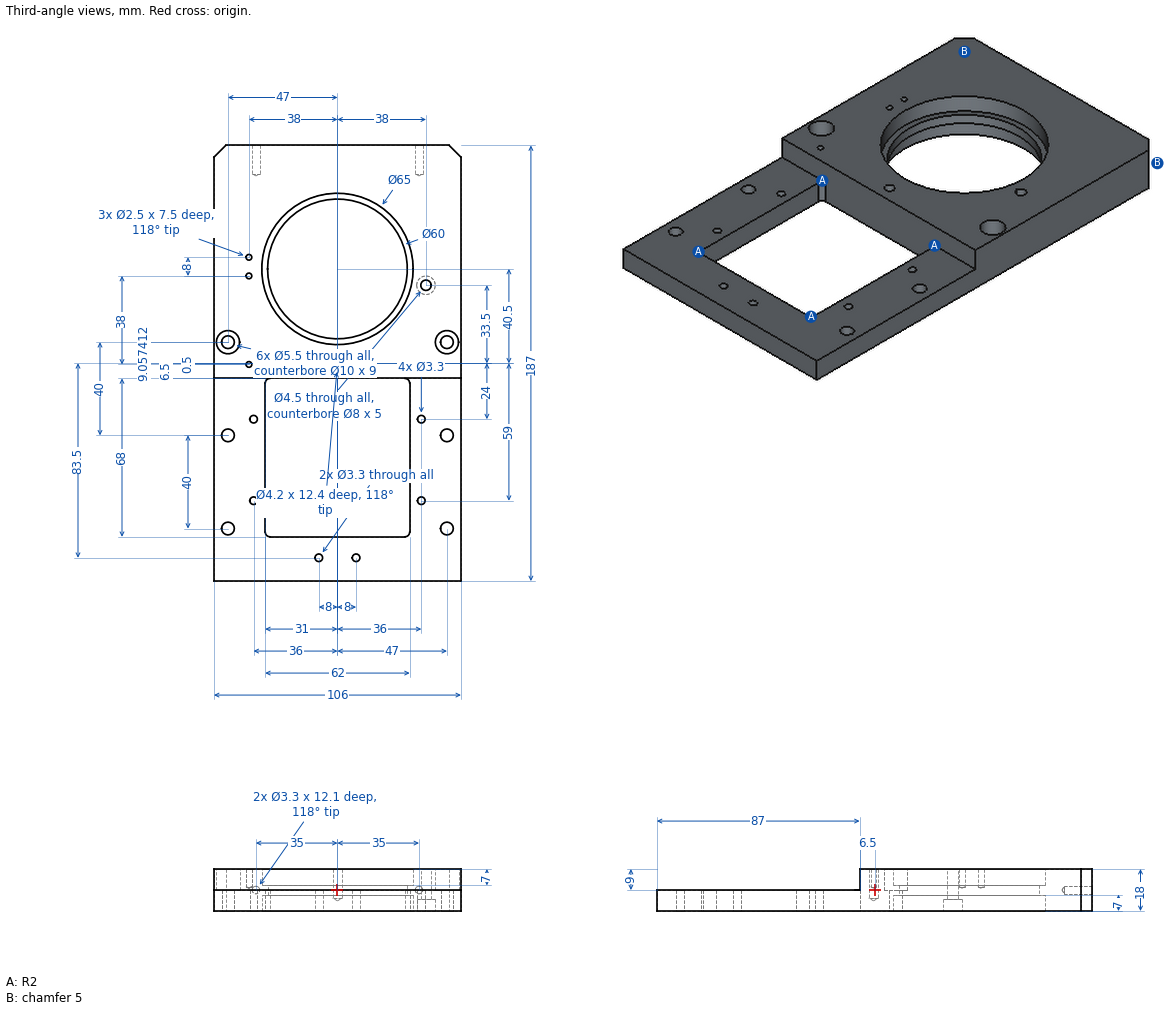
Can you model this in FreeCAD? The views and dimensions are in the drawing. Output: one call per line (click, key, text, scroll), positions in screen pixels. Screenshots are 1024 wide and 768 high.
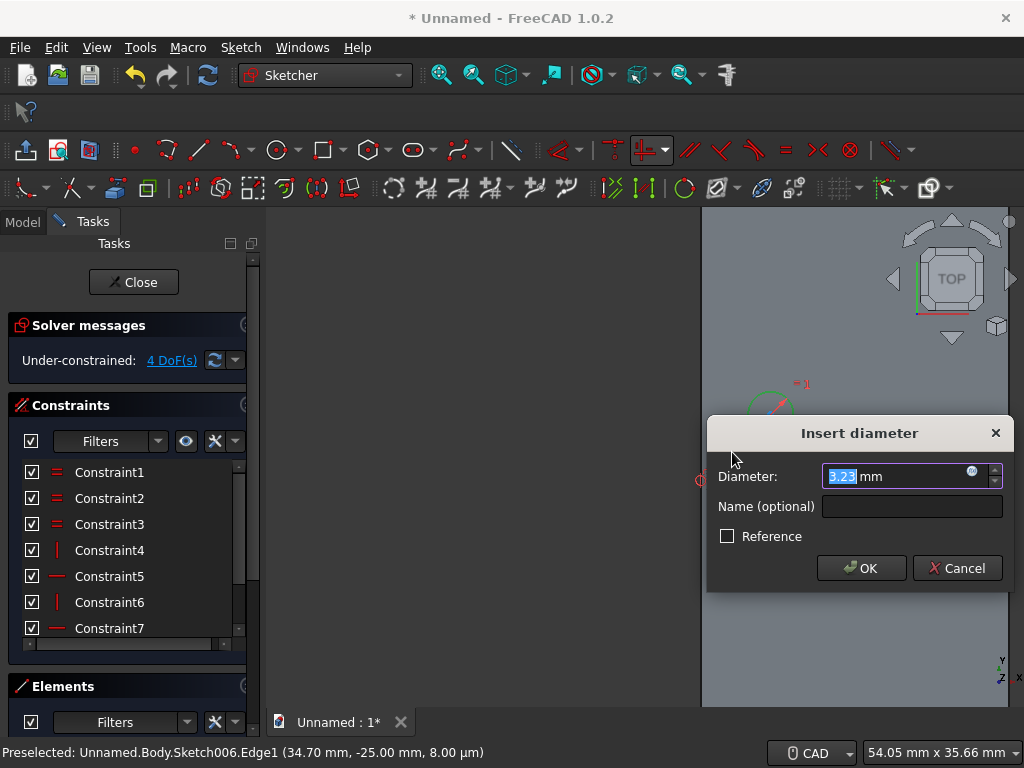
text(3.3)
key(Return)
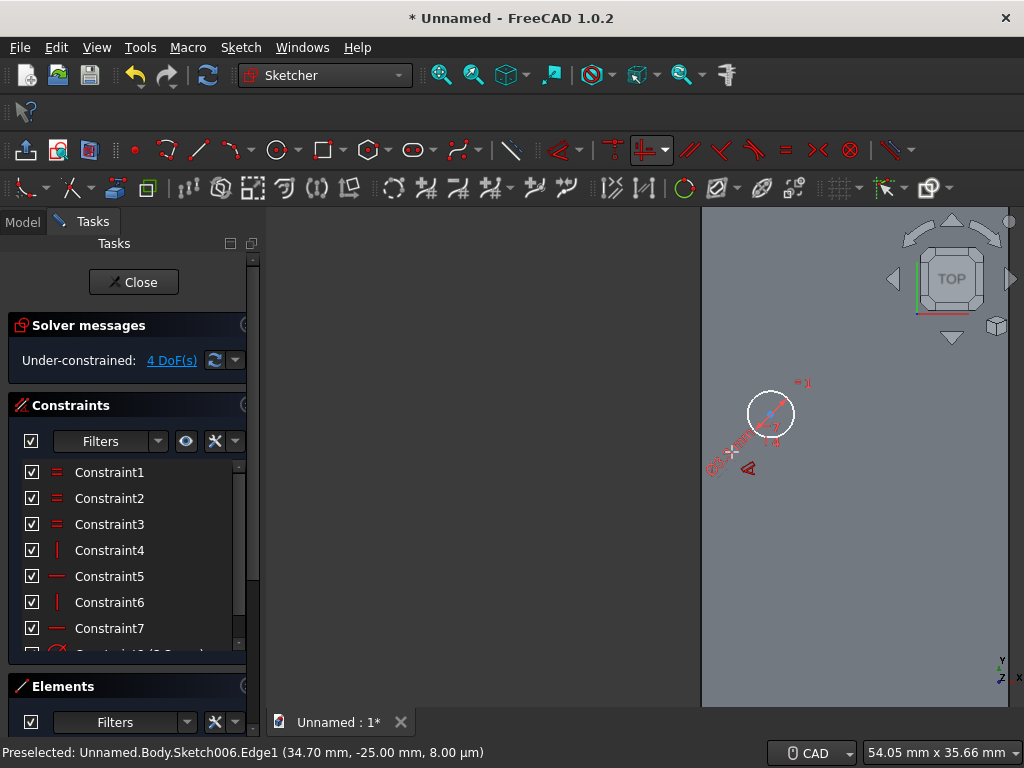
click(771, 414)
click(532, 448)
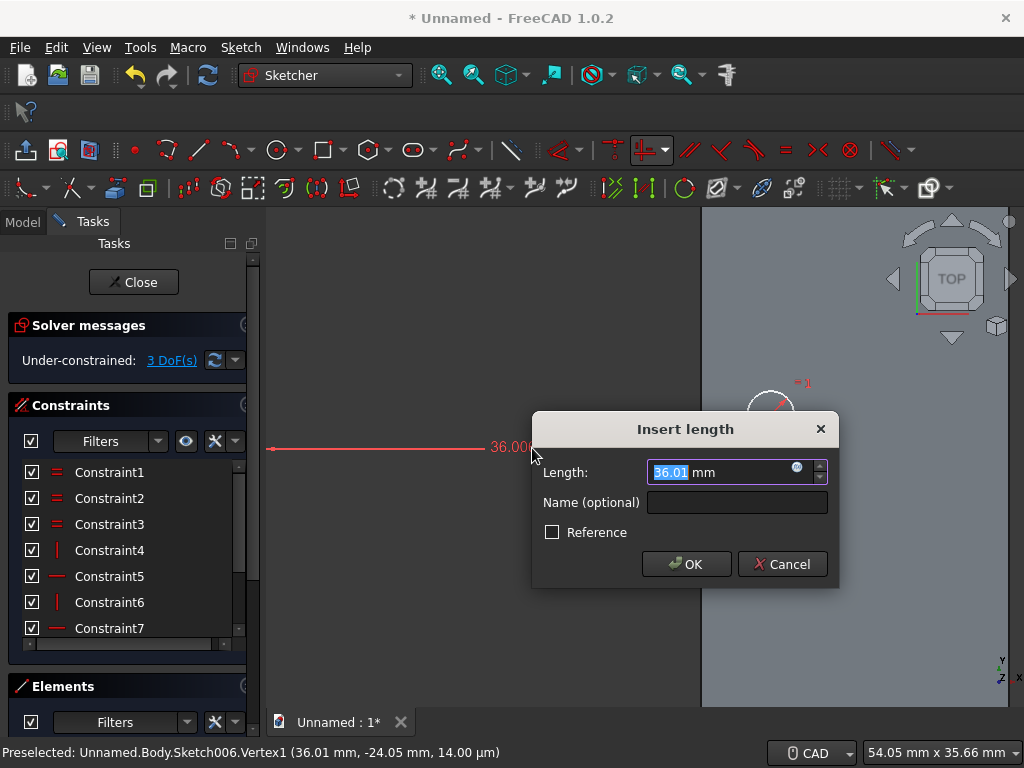
text(36)
key(Return)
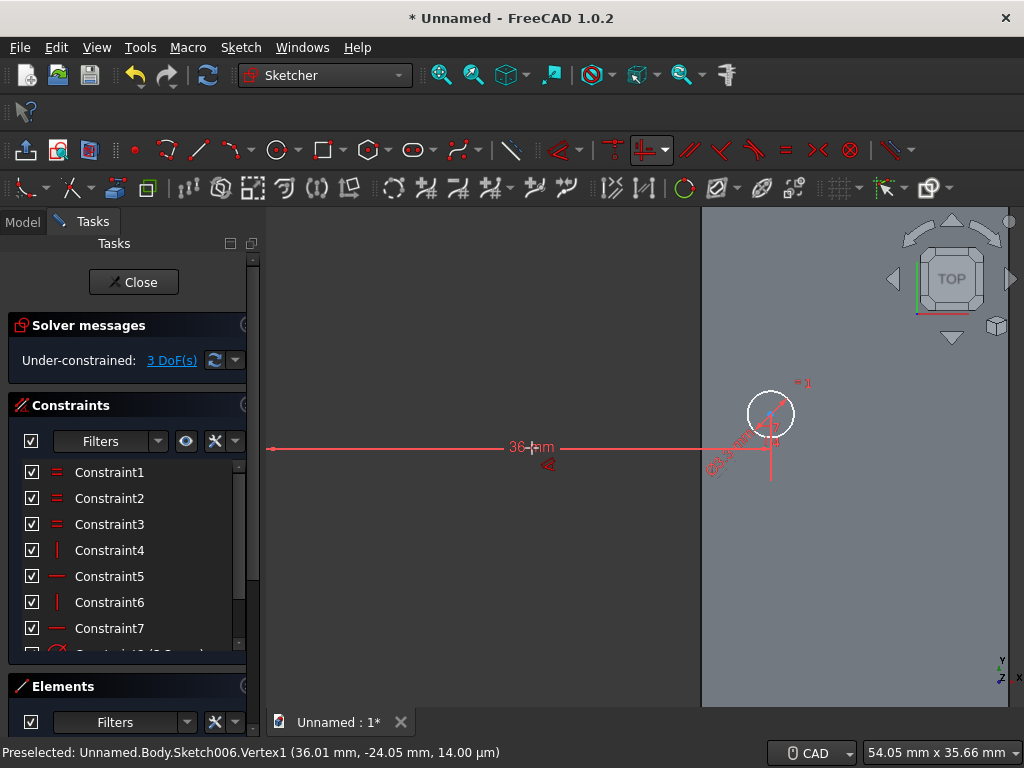
click(771, 414)
click(805, 325)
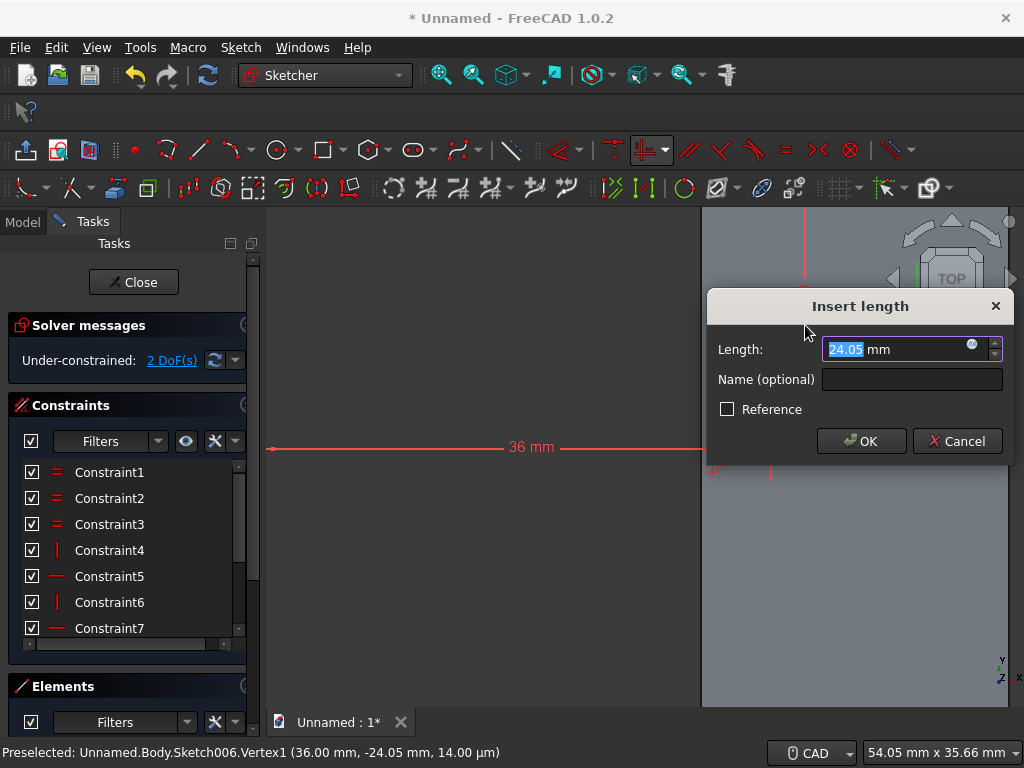
text(24)
key(Return)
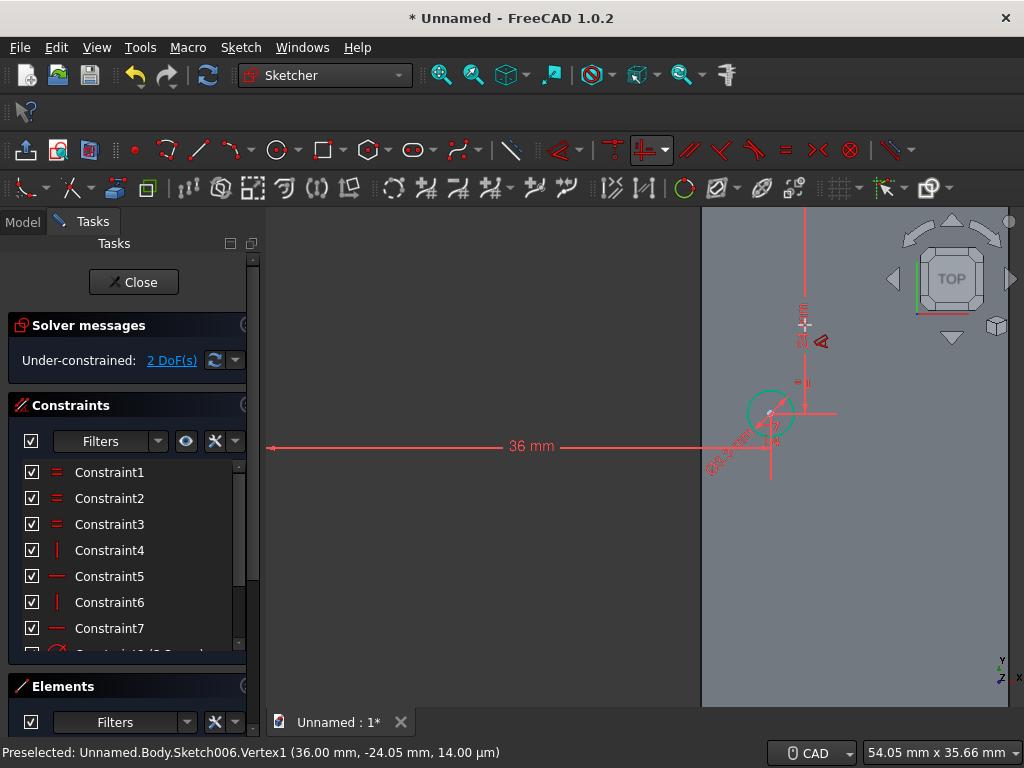
scroll(757, 431, down, 5)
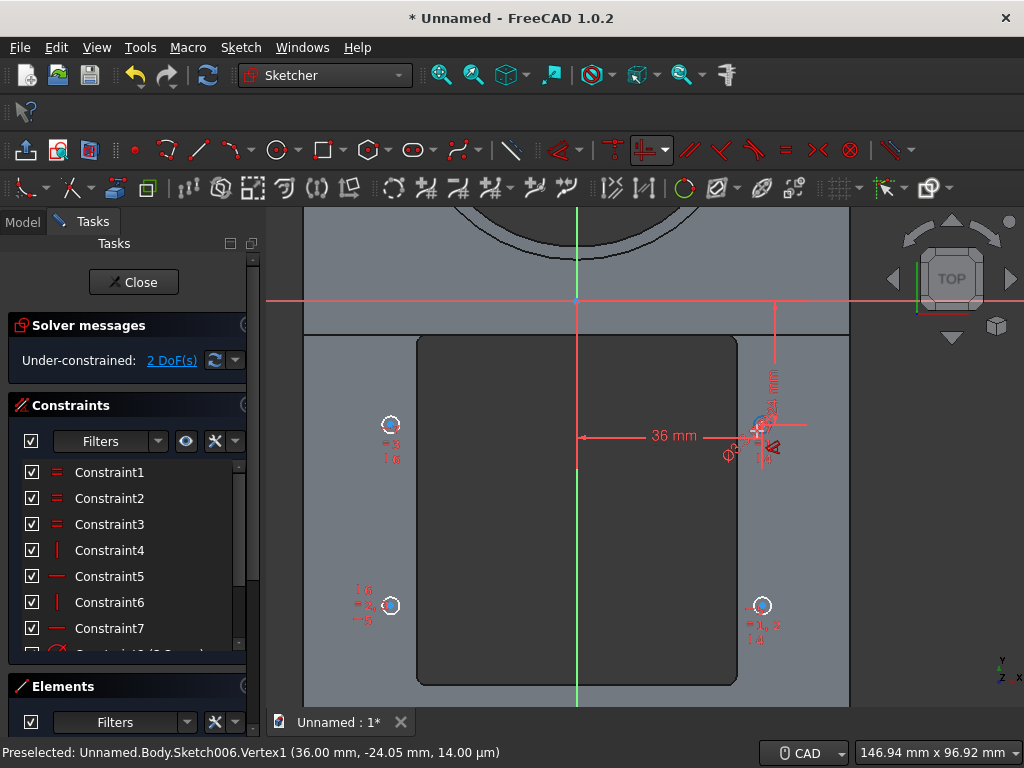
click(762, 606)
click(796, 524)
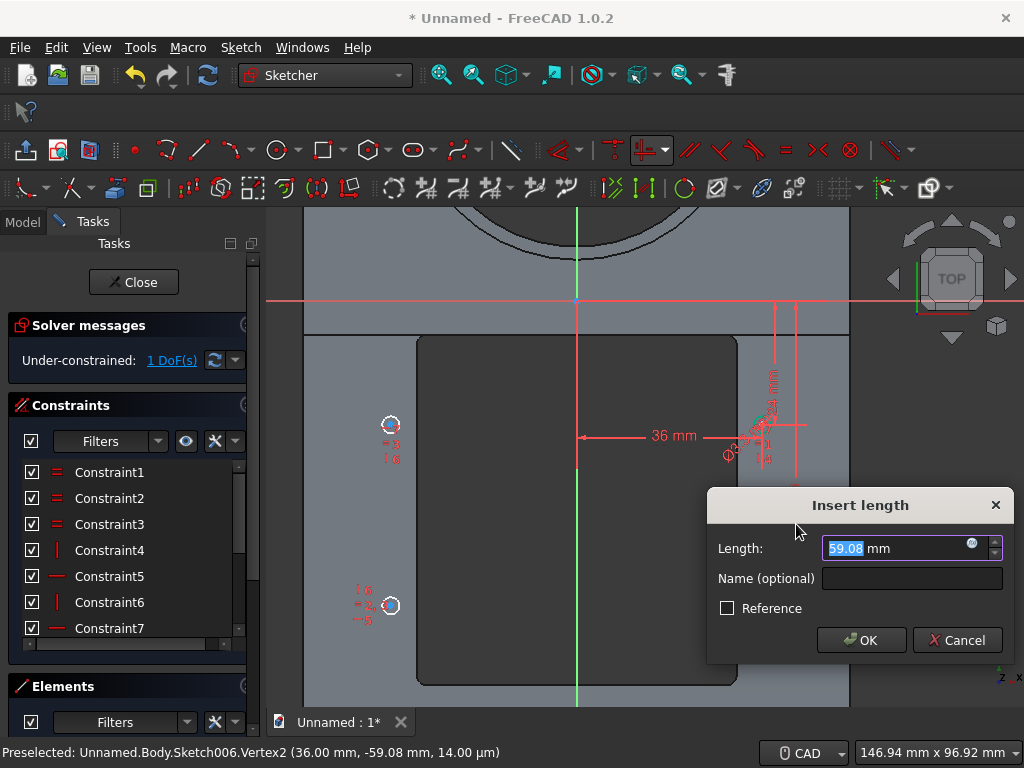
text(59)
key(Return)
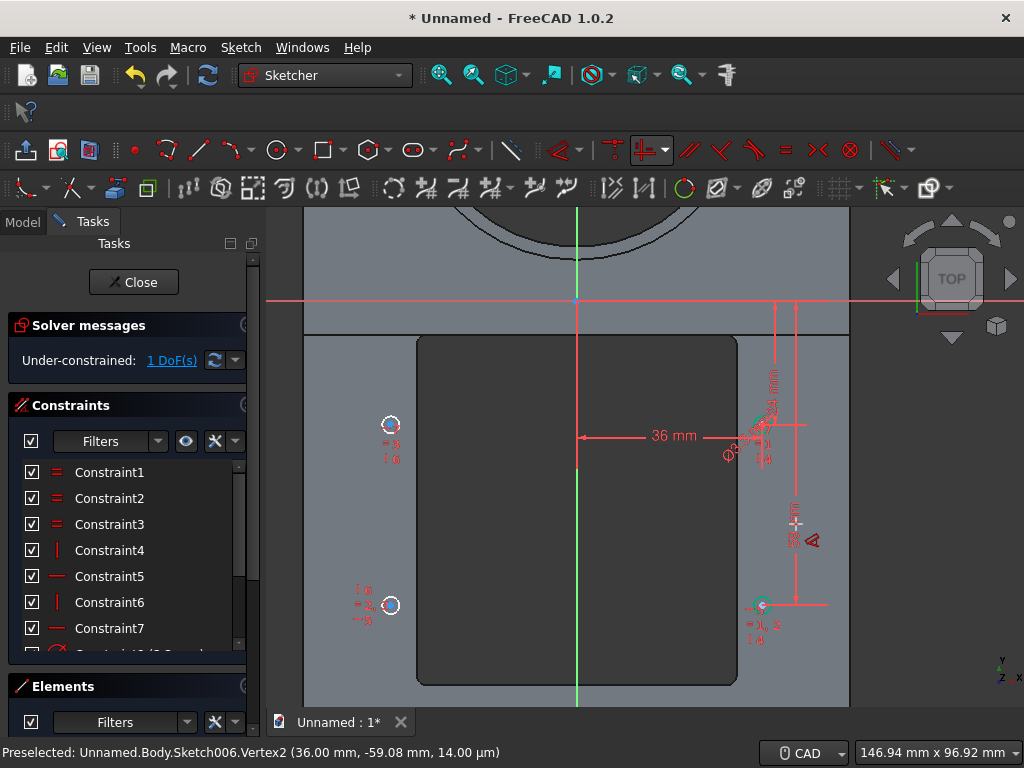
click(391, 605)
click(484, 267)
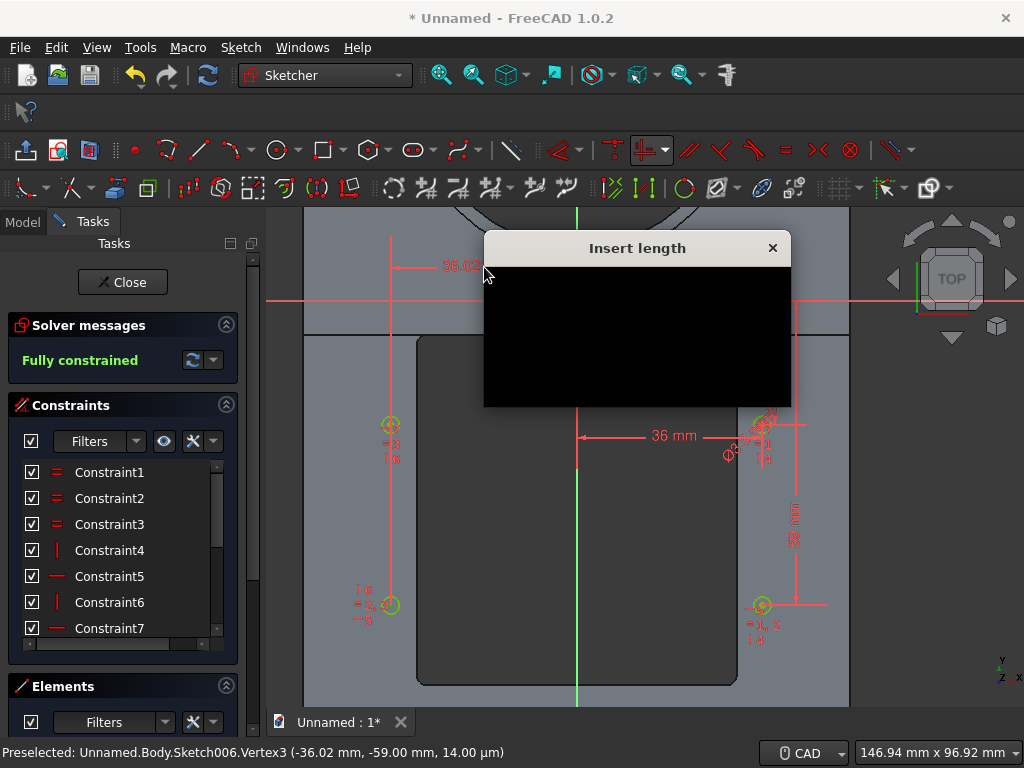
text(36)
key(Return)
key(Escape)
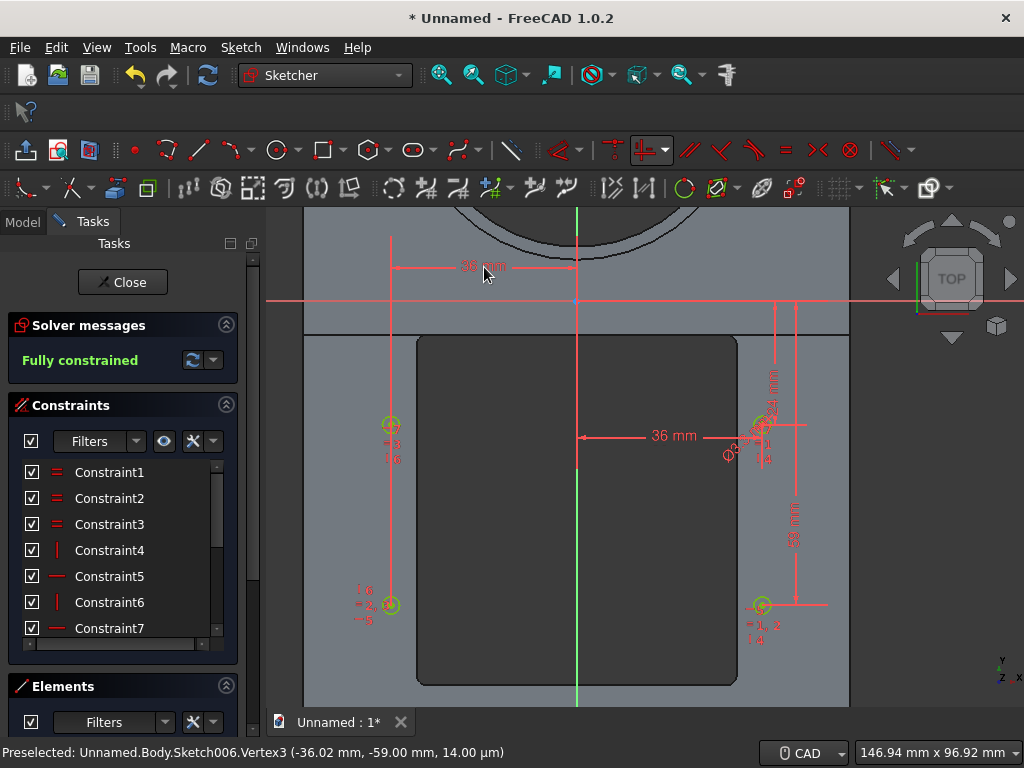
click(123, 282)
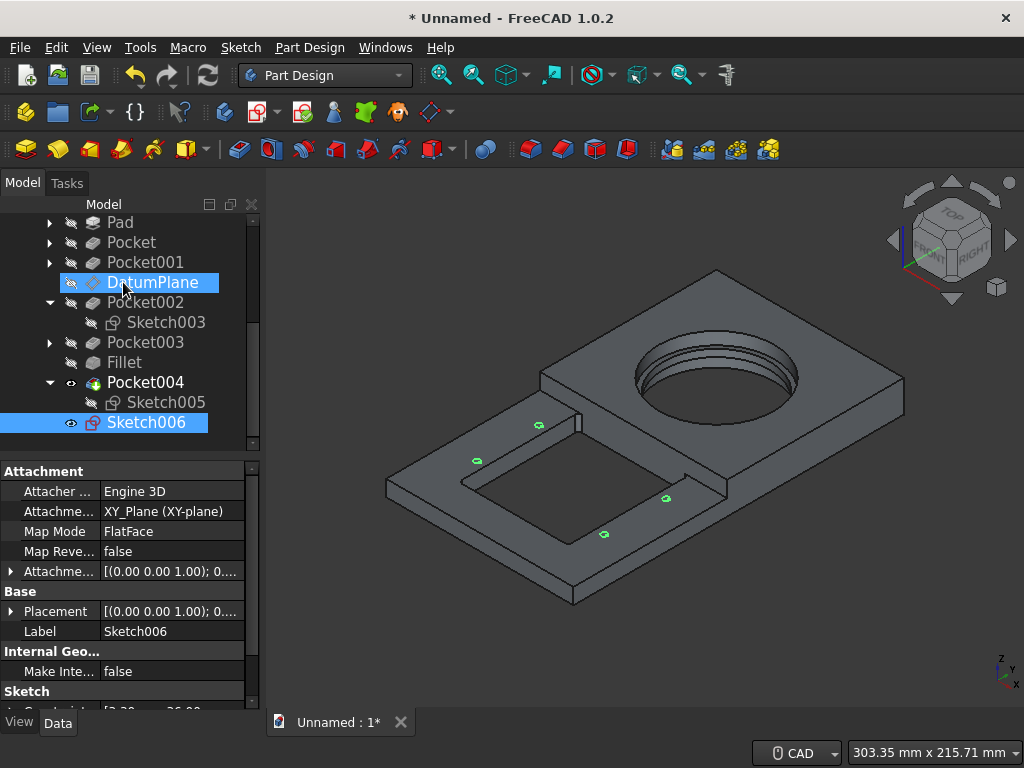
click(240, 150)